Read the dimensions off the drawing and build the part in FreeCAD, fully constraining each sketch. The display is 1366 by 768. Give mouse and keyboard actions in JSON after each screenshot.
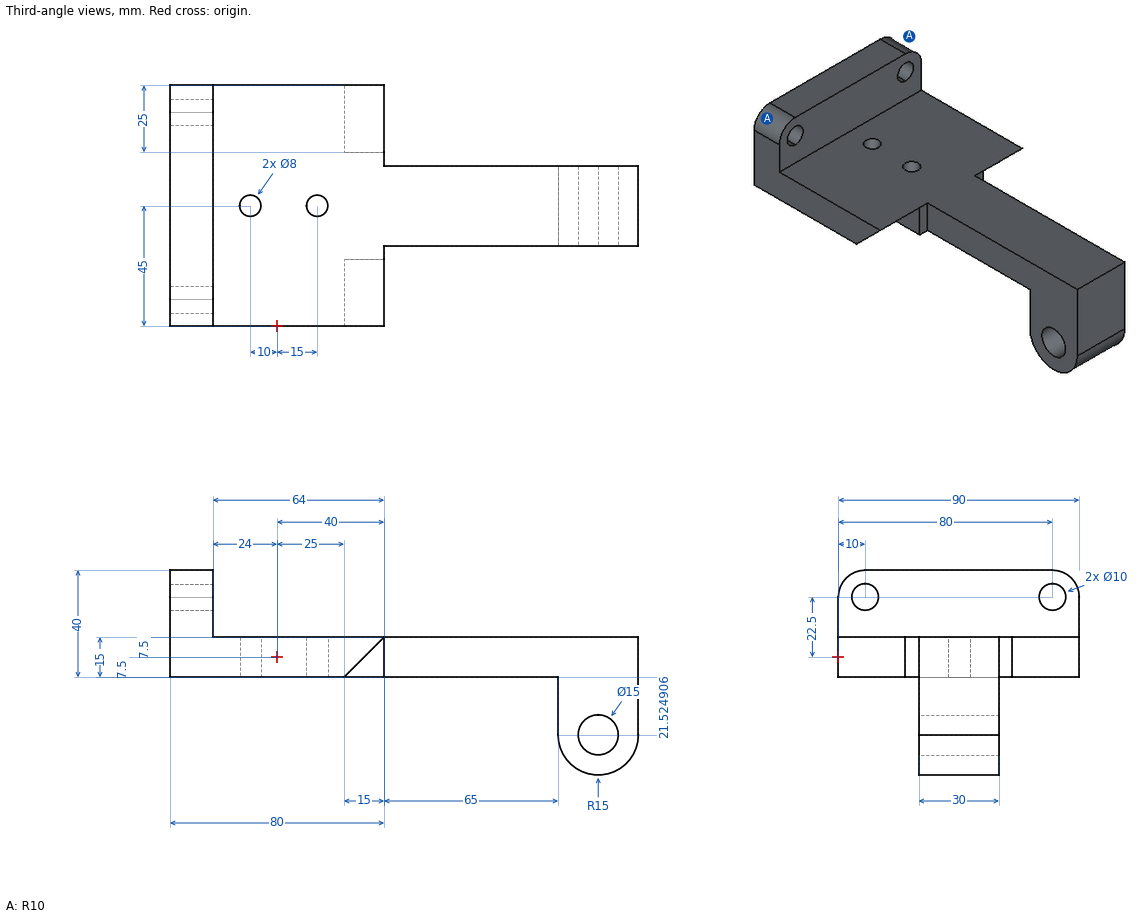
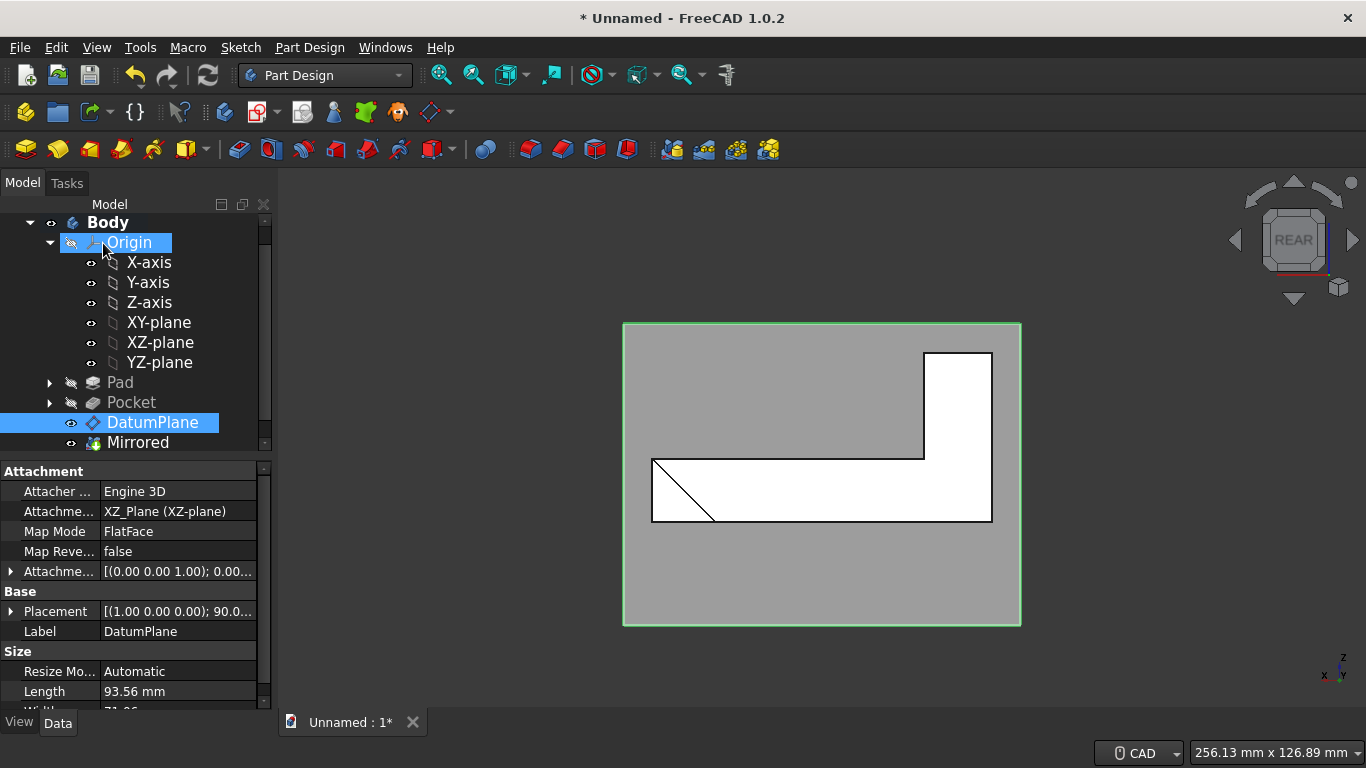
{"action": "left_click", "coordinate": [116, 423]}
{"action": "key", "text": "space"}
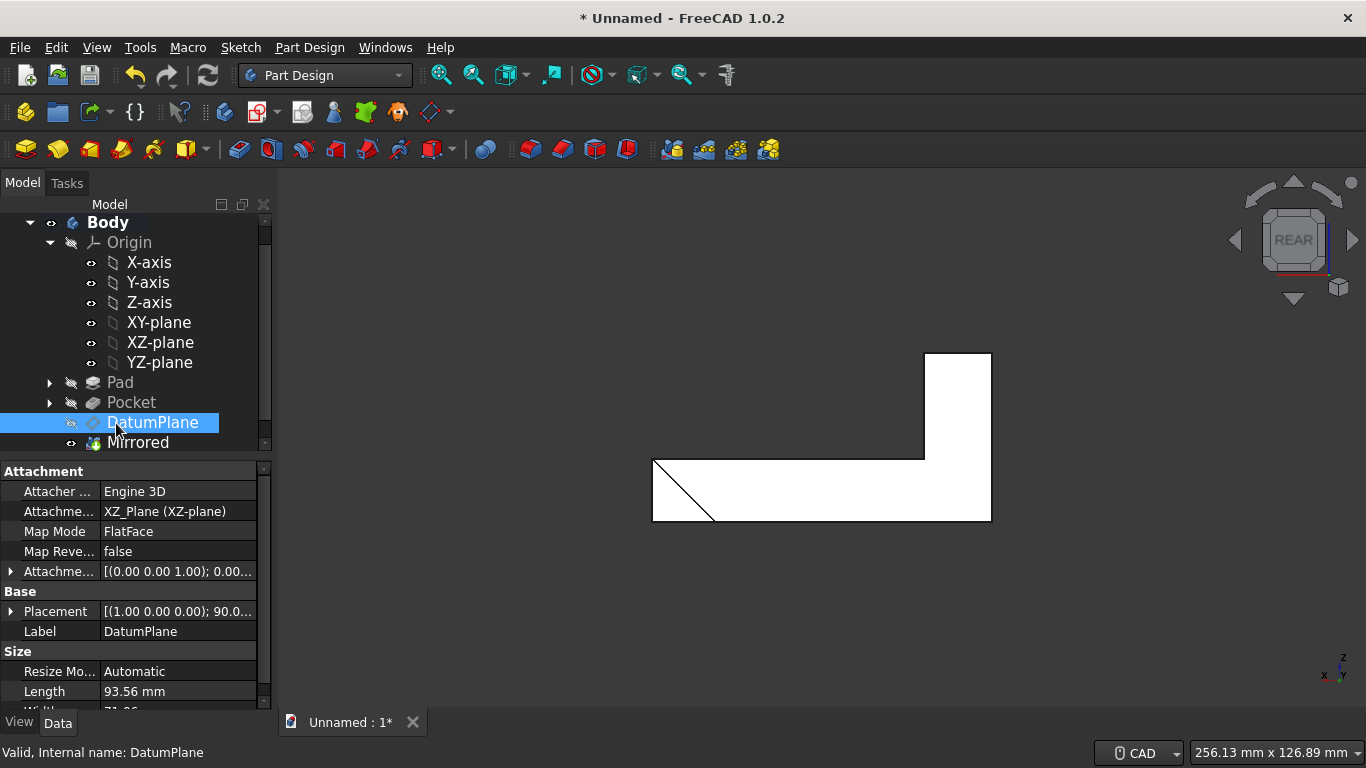
{"action": "left_click", "coordinate": [442, 76]}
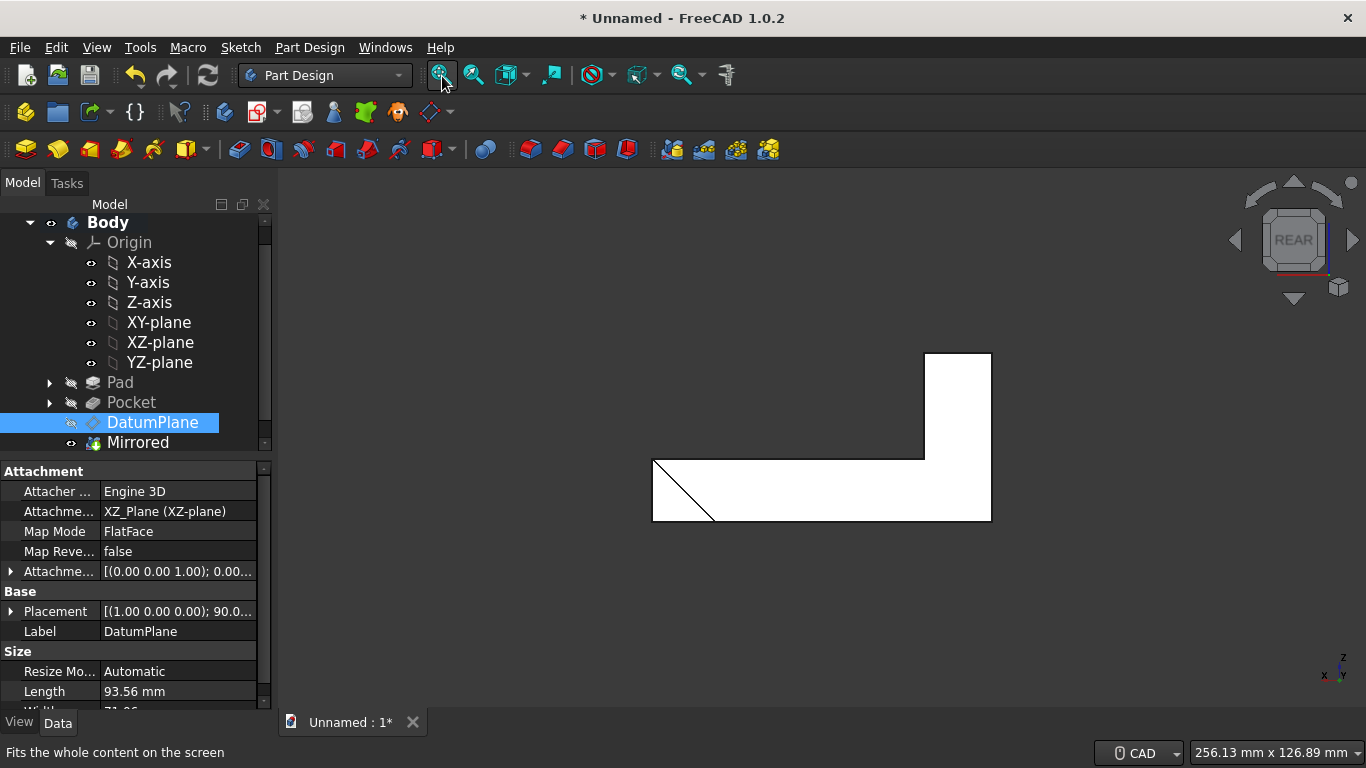
{"action": "left_click", "coordinate": [136, 343]}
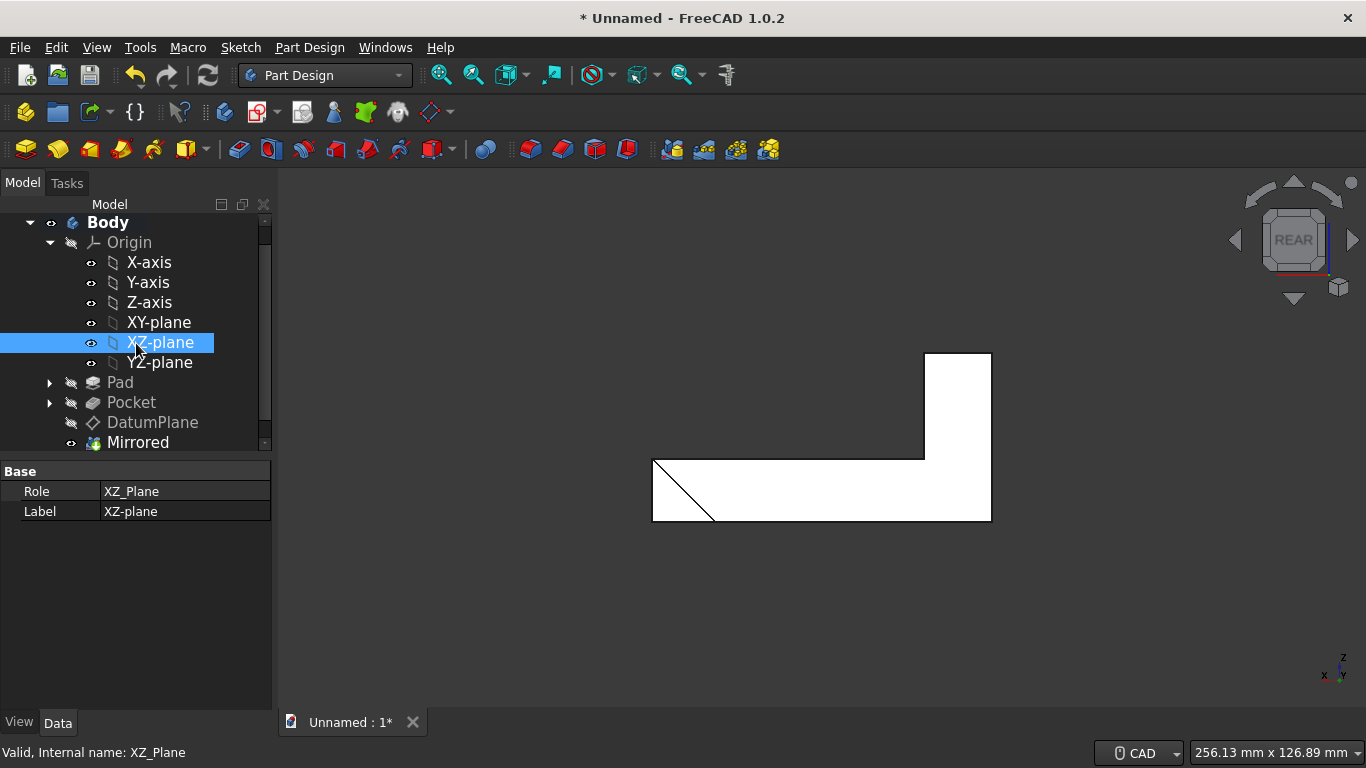
{"action": "left_click", "coordinate": [430, 112]}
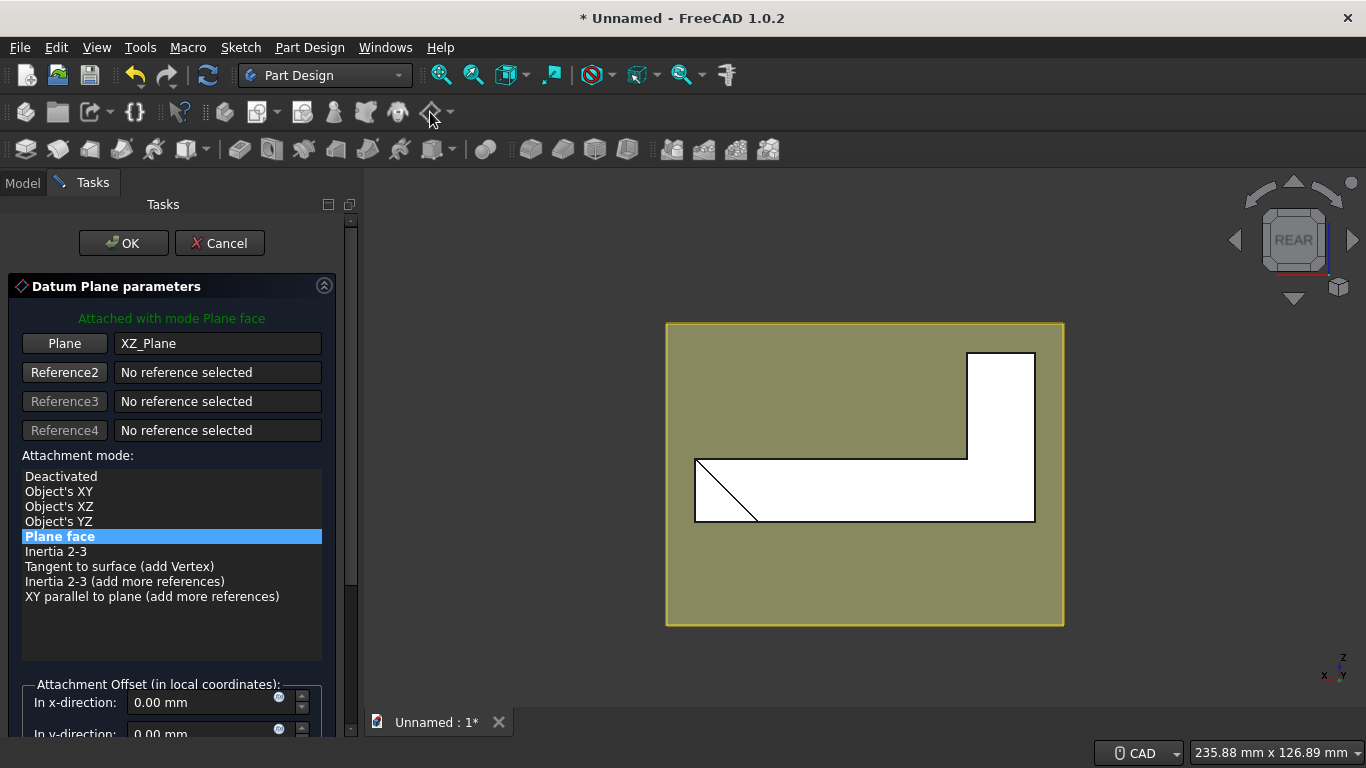
{"action": "scroll", "coordinate": [351, 475], "scroll_direction": "down", "scroll_amount": 2}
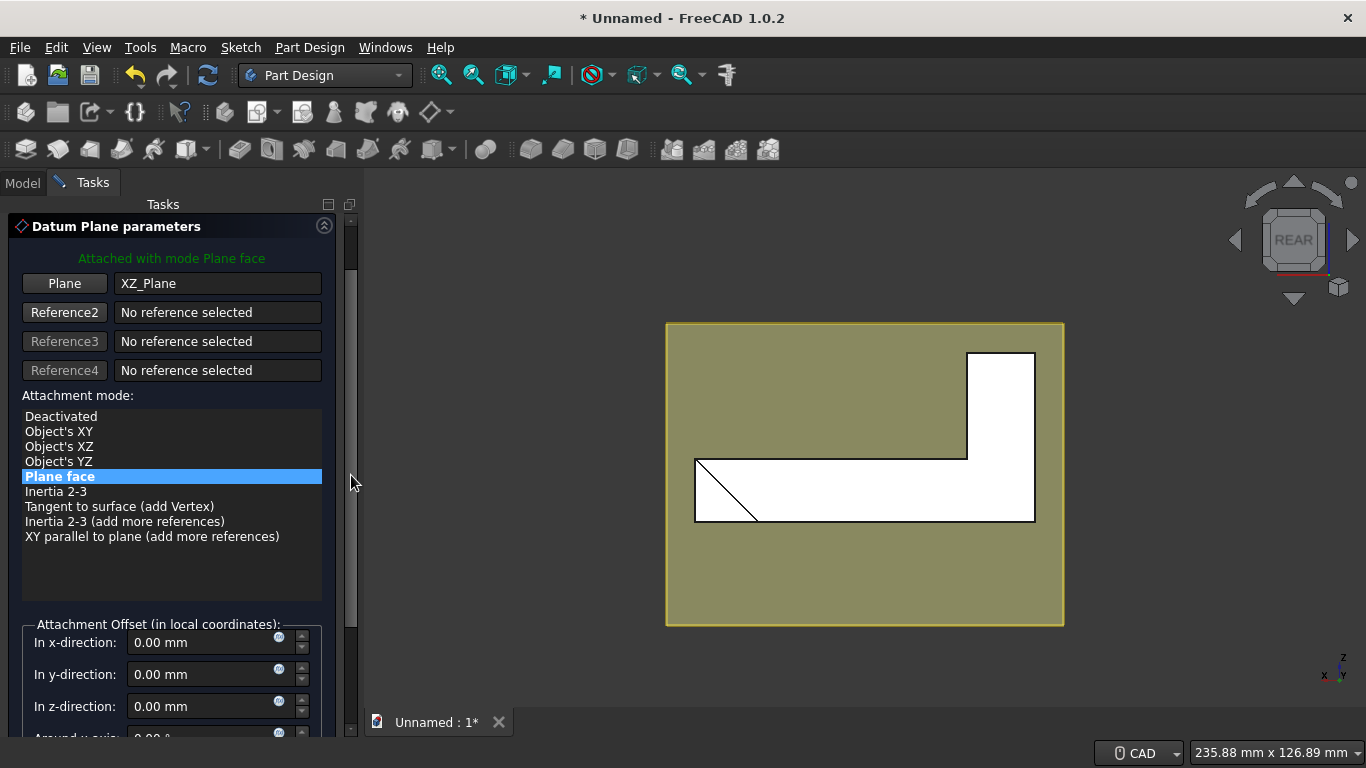
{"action": "triple_click", "coordinate": [210, 646]}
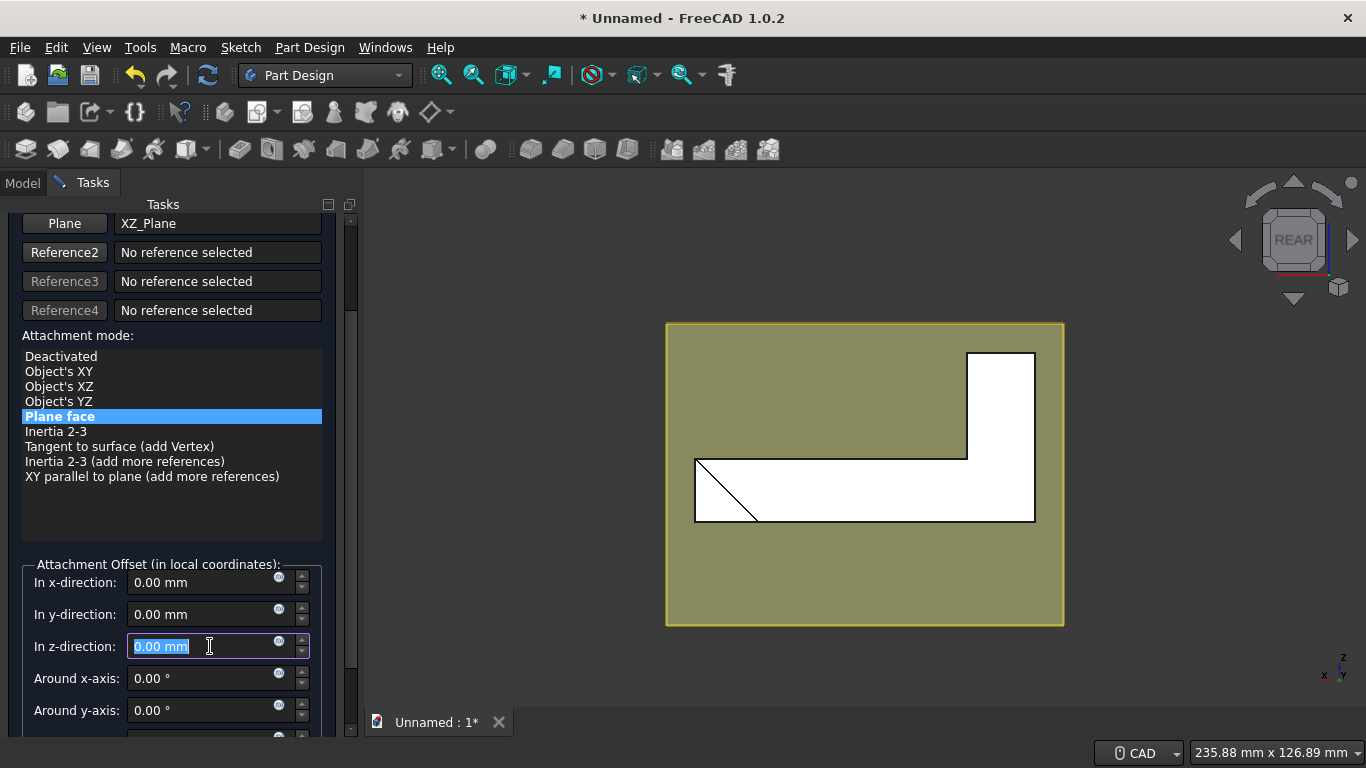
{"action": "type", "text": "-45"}
{"action": "key", "text": "Tab"}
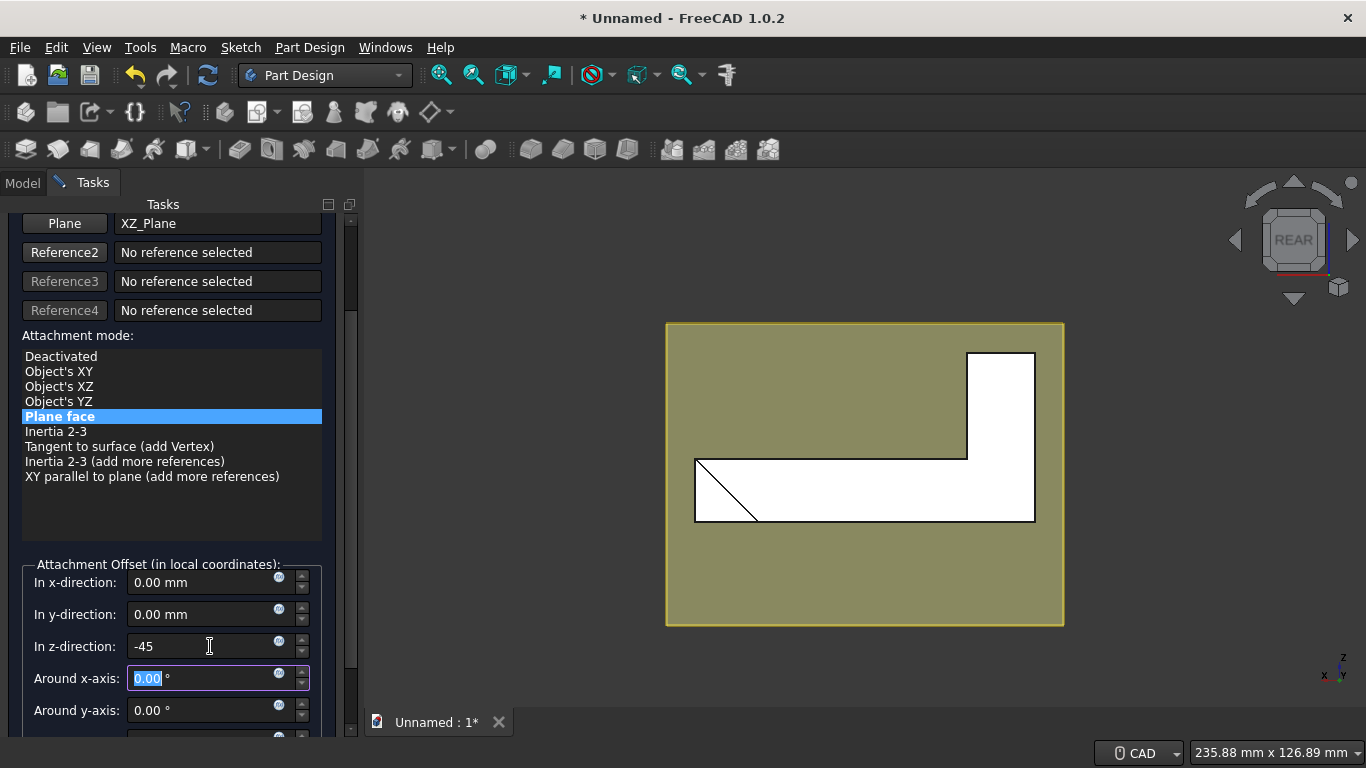
{"action": "scroll", "coordinate": [351, 475], "scroll_direction": "up", "scroll_amount": 3}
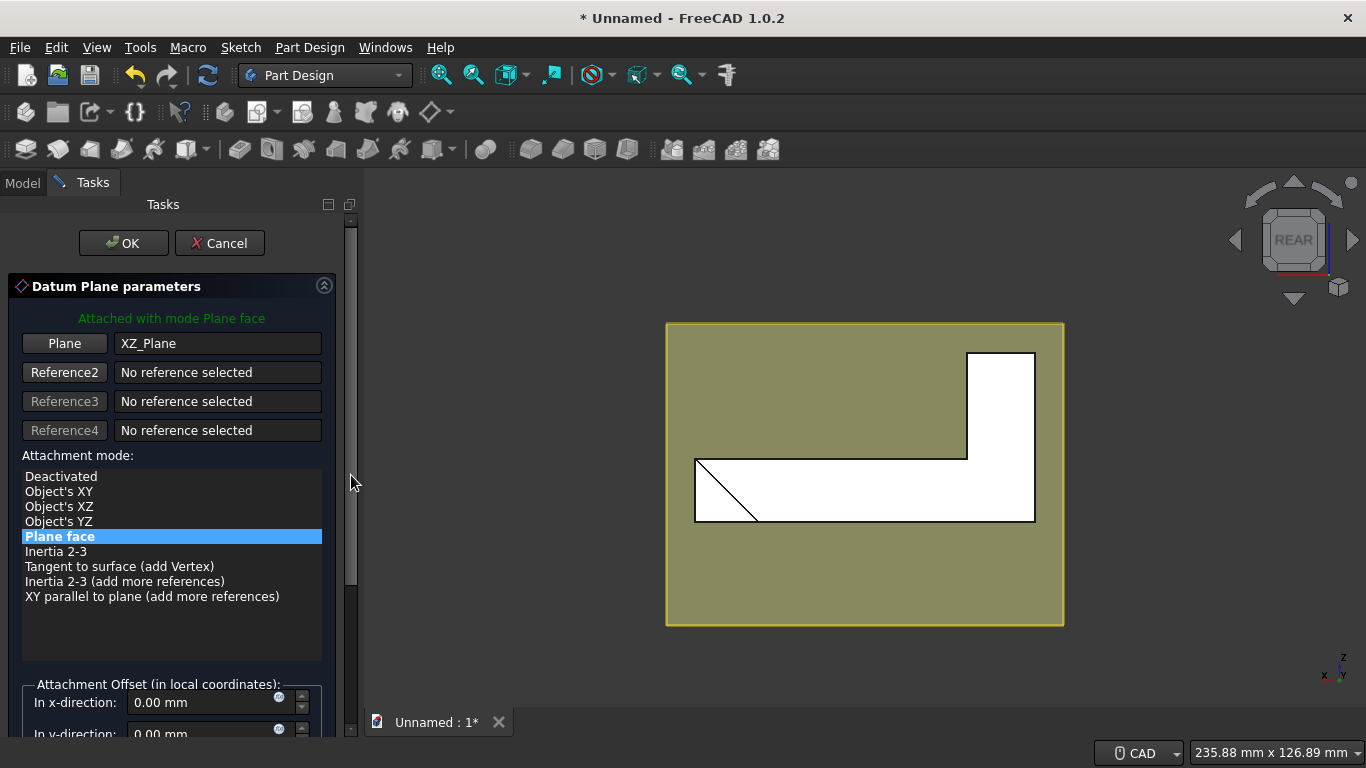
{"action": "left_click", "coordinate": [124, 243]}